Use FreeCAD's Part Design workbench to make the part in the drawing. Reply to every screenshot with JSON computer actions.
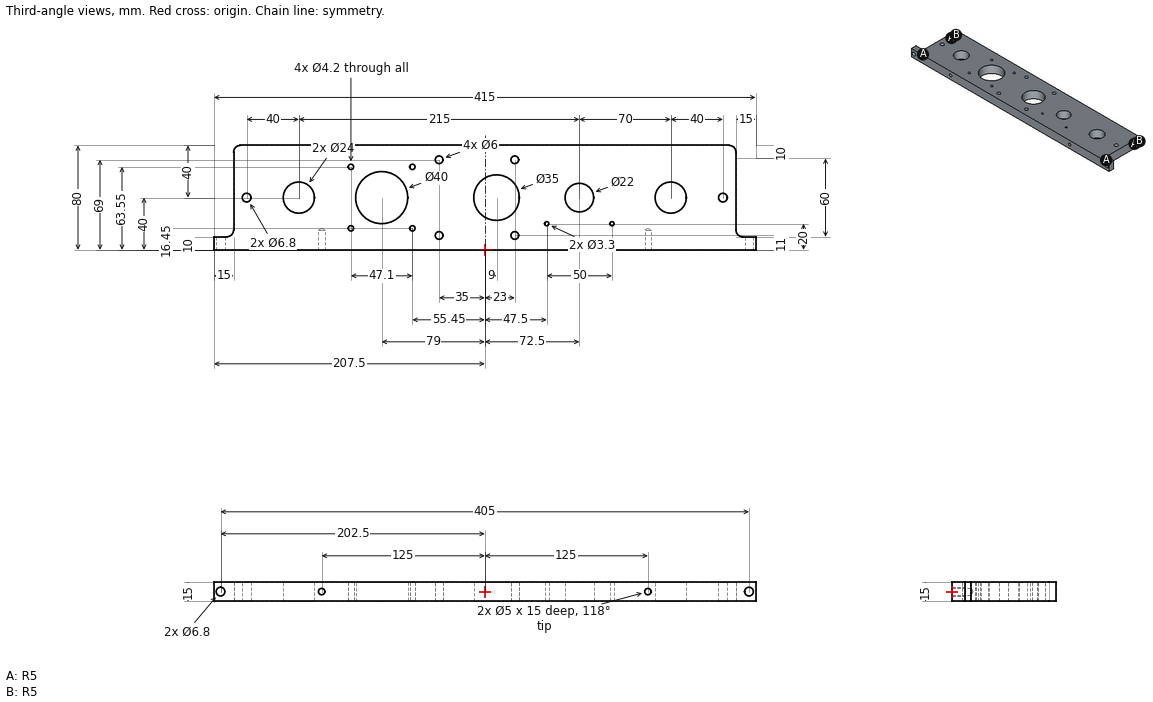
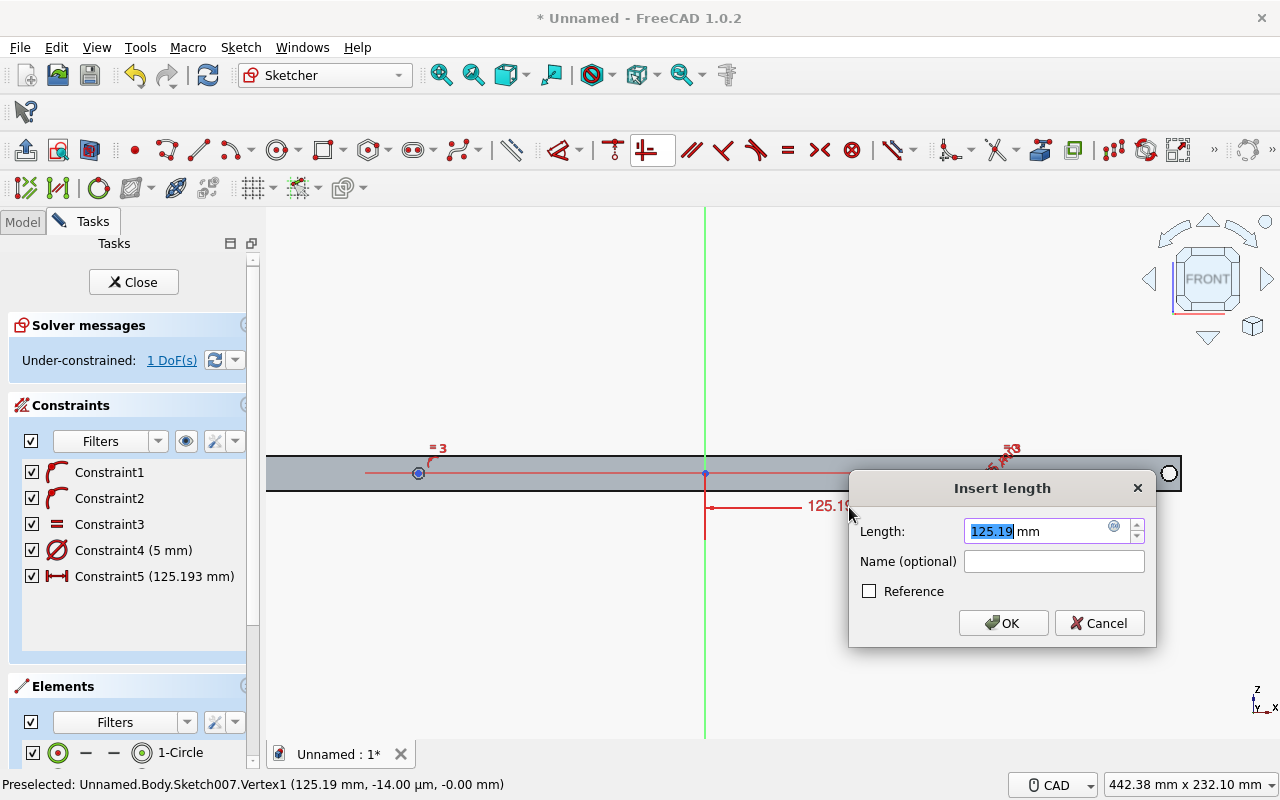
{"action": "type", "text": "125"}
{"action": "key", "text": "Return"}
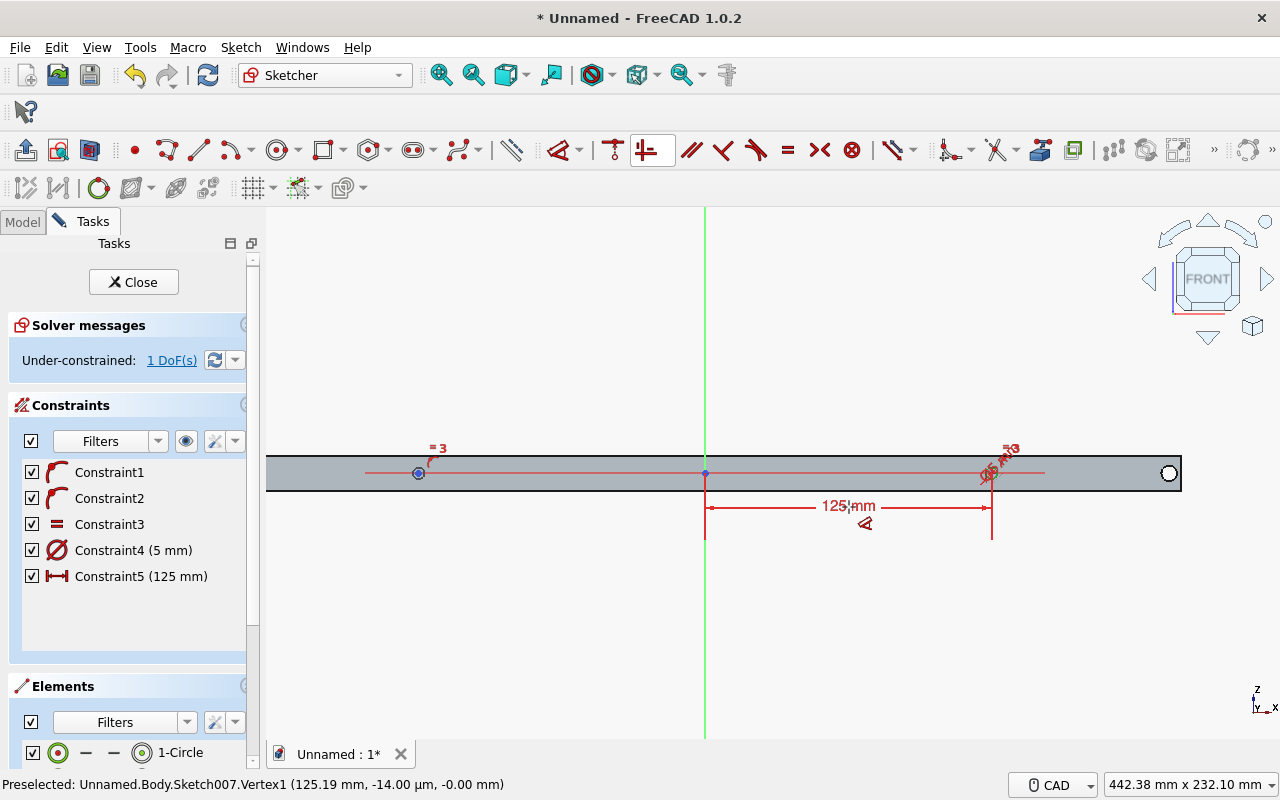
{"action": "left_click", "coordinate": [419, 473]}
{"action": "left_click", "coordinate": [562, 507]}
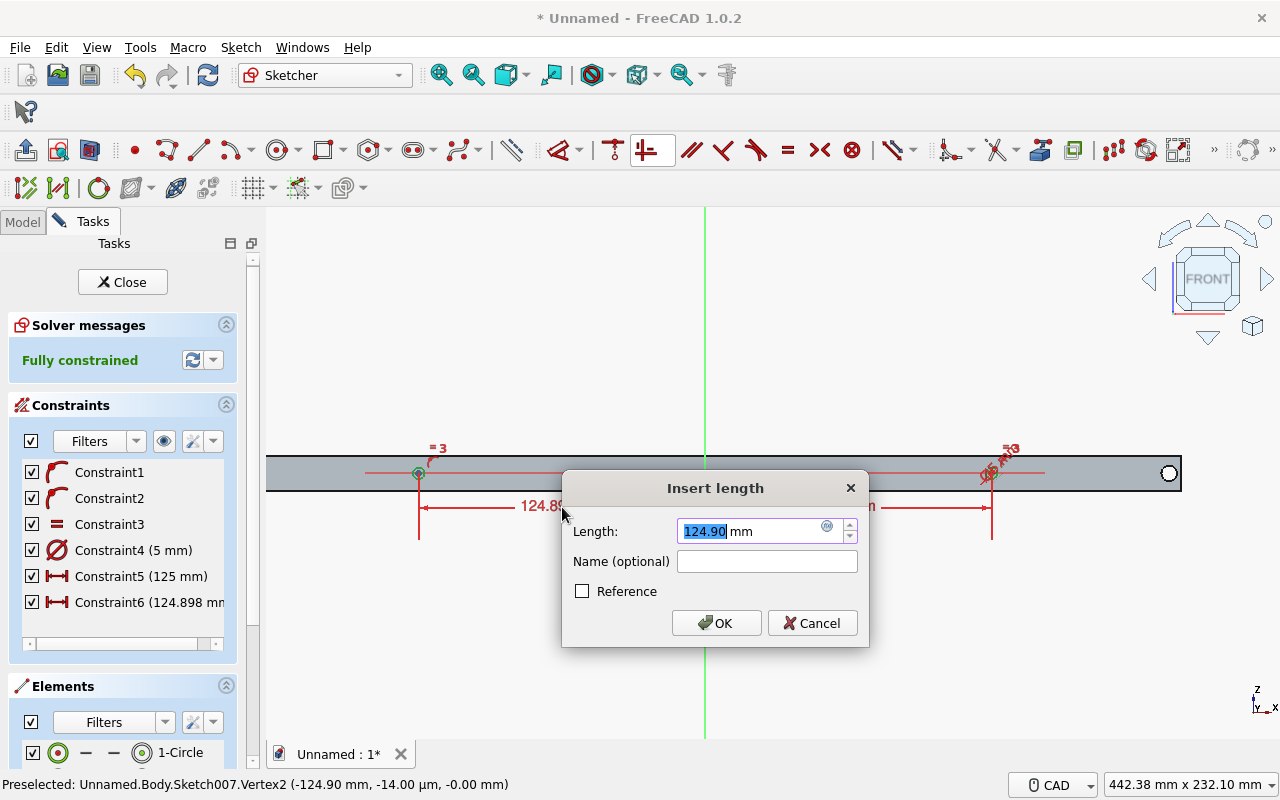
{"action": "type", "text": "125"}
{"action": "key", "text": "Return"}
{"action": "key", "text": "Escape"}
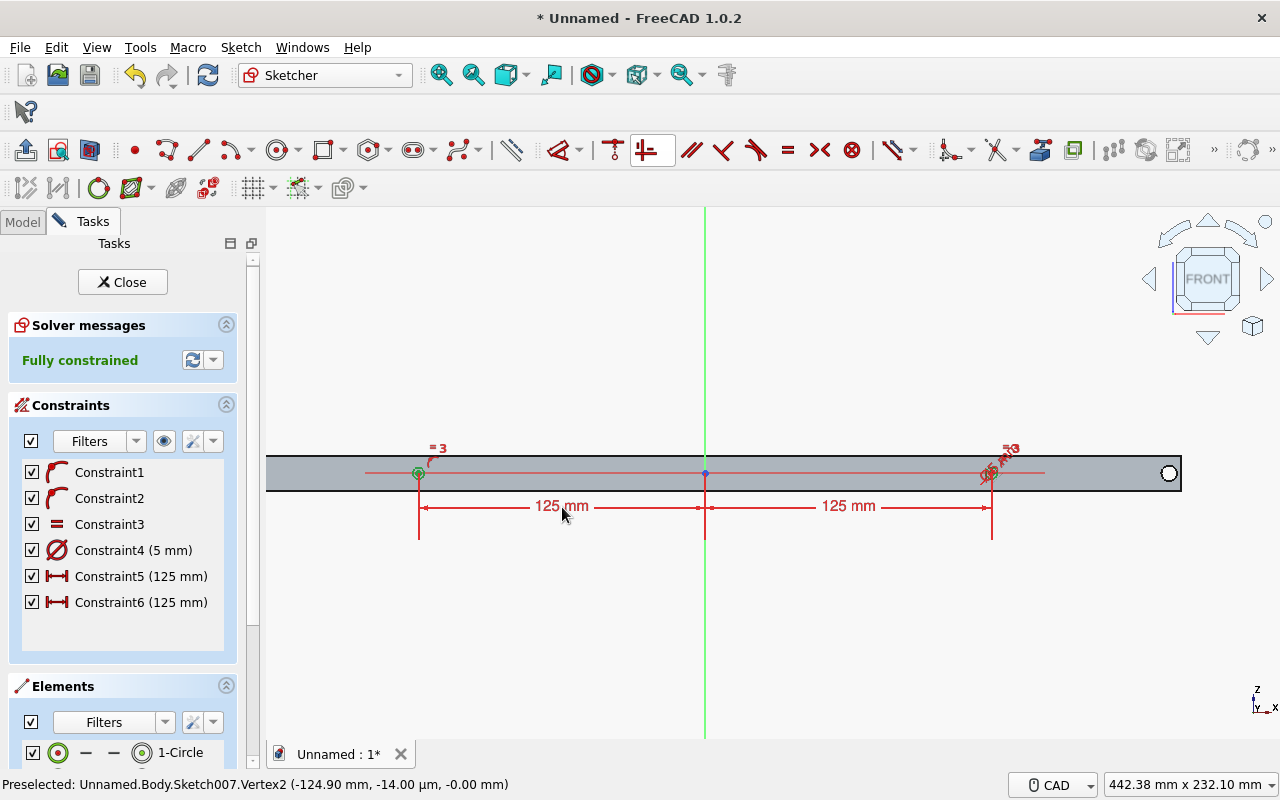
{"action": "left_click", "coordinate": [123, 282]}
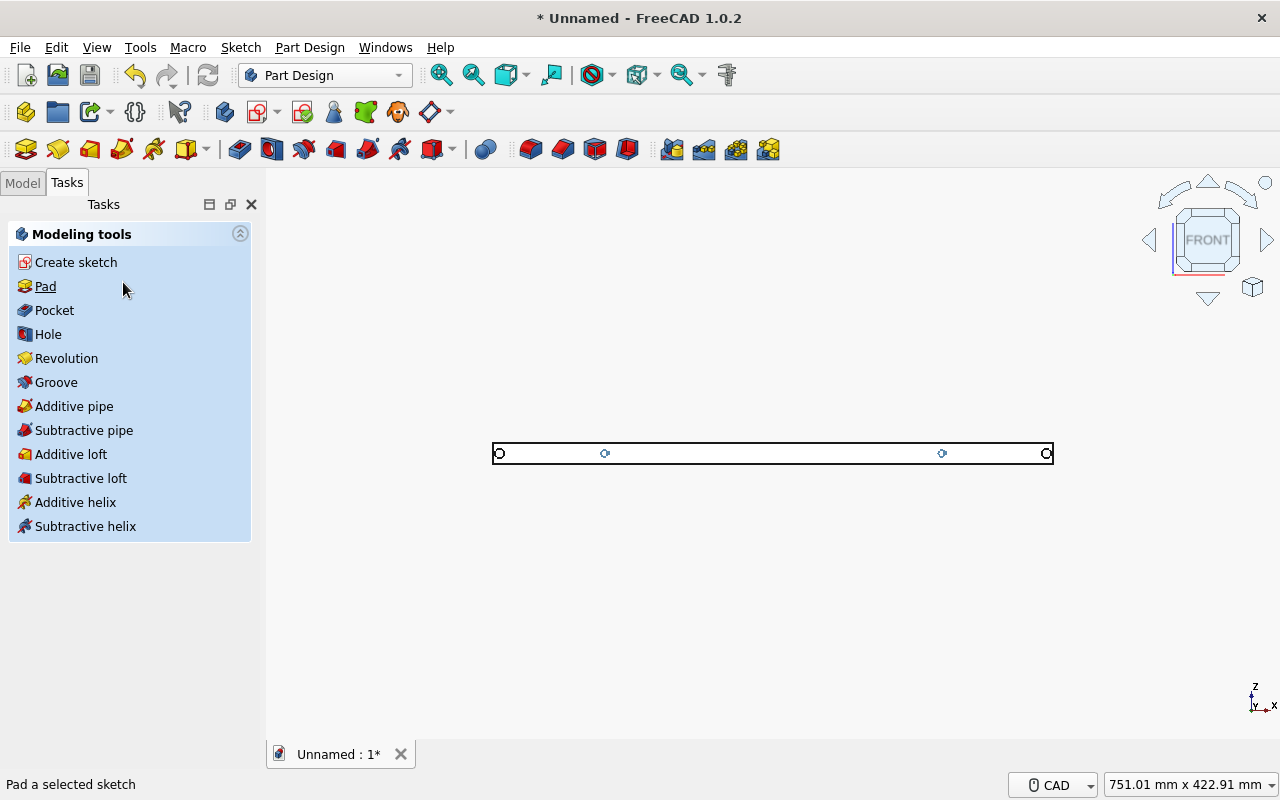
{"action": "left_click", "coordinate": [272, 150]}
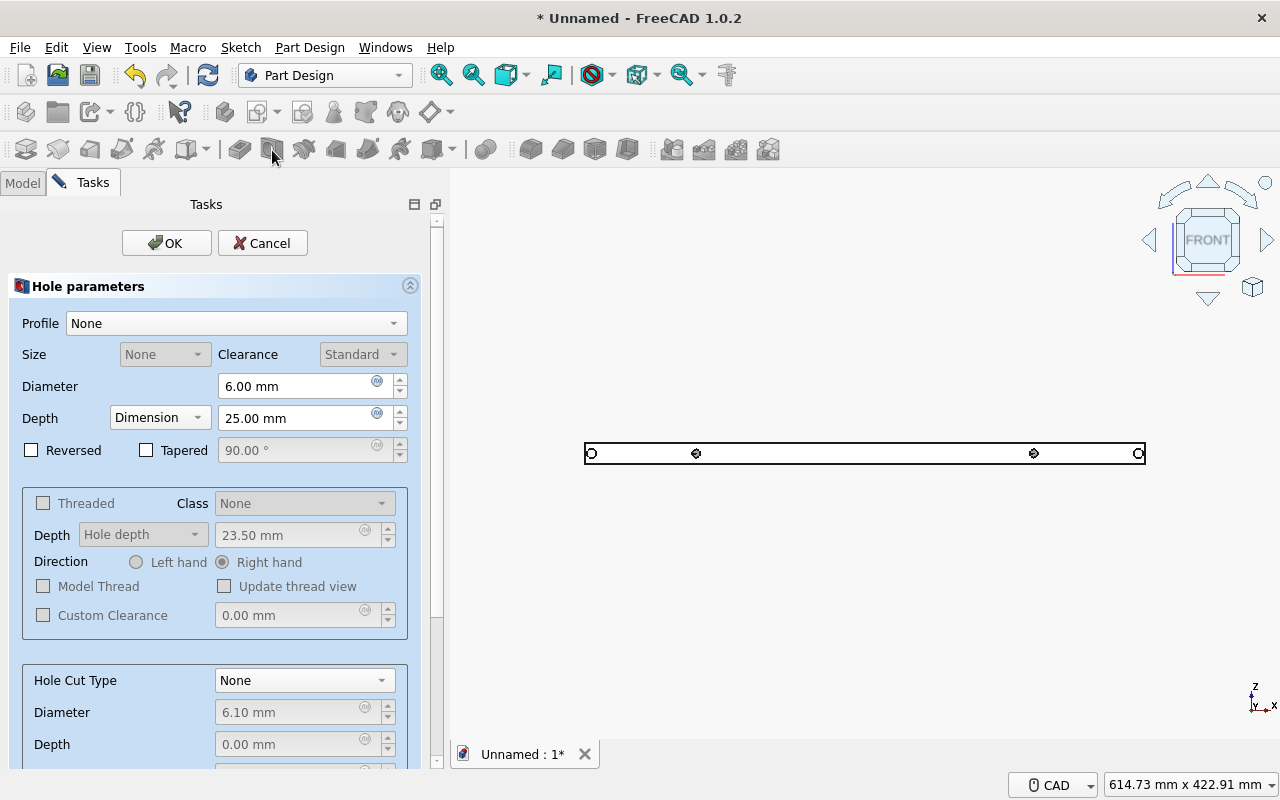
{"action": "triple_click", "coordinate": [305, 386]}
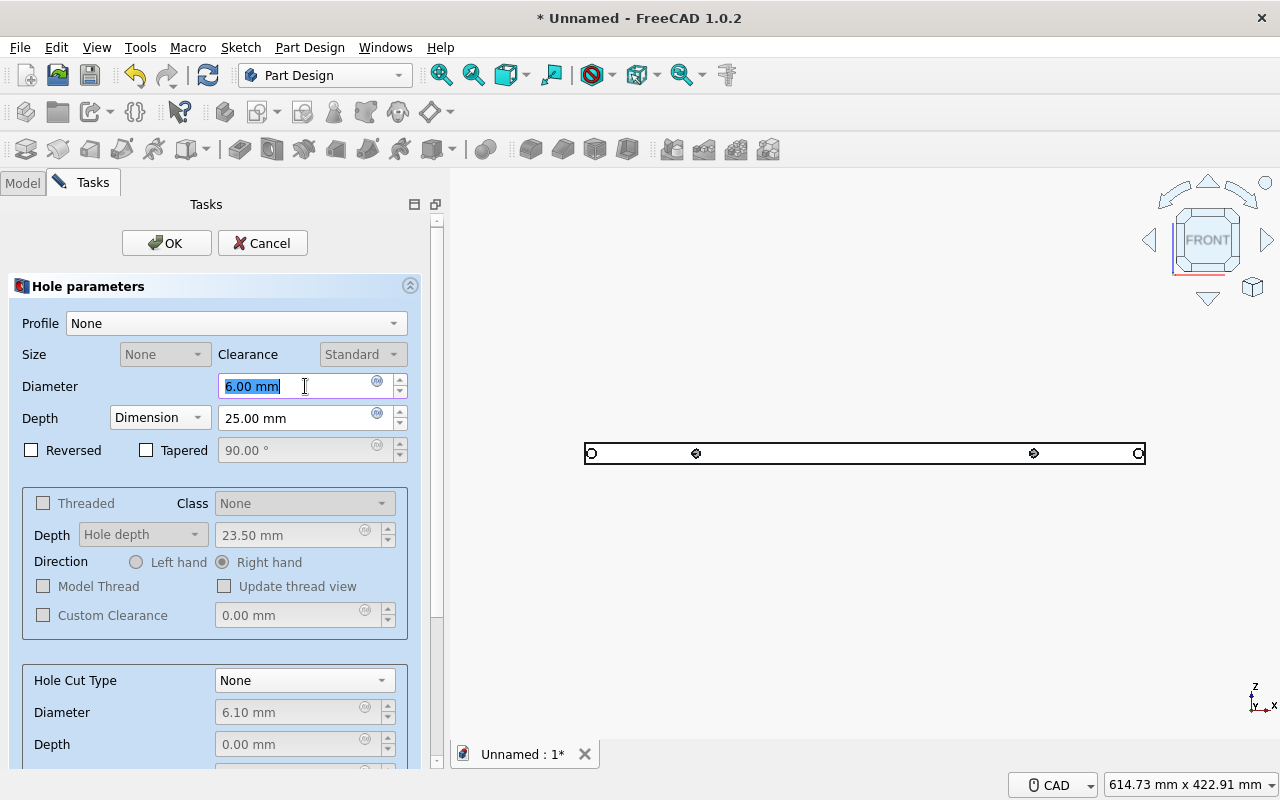
{"action": "type", "text": "5"}
{"action": "key", "text": "Tab"}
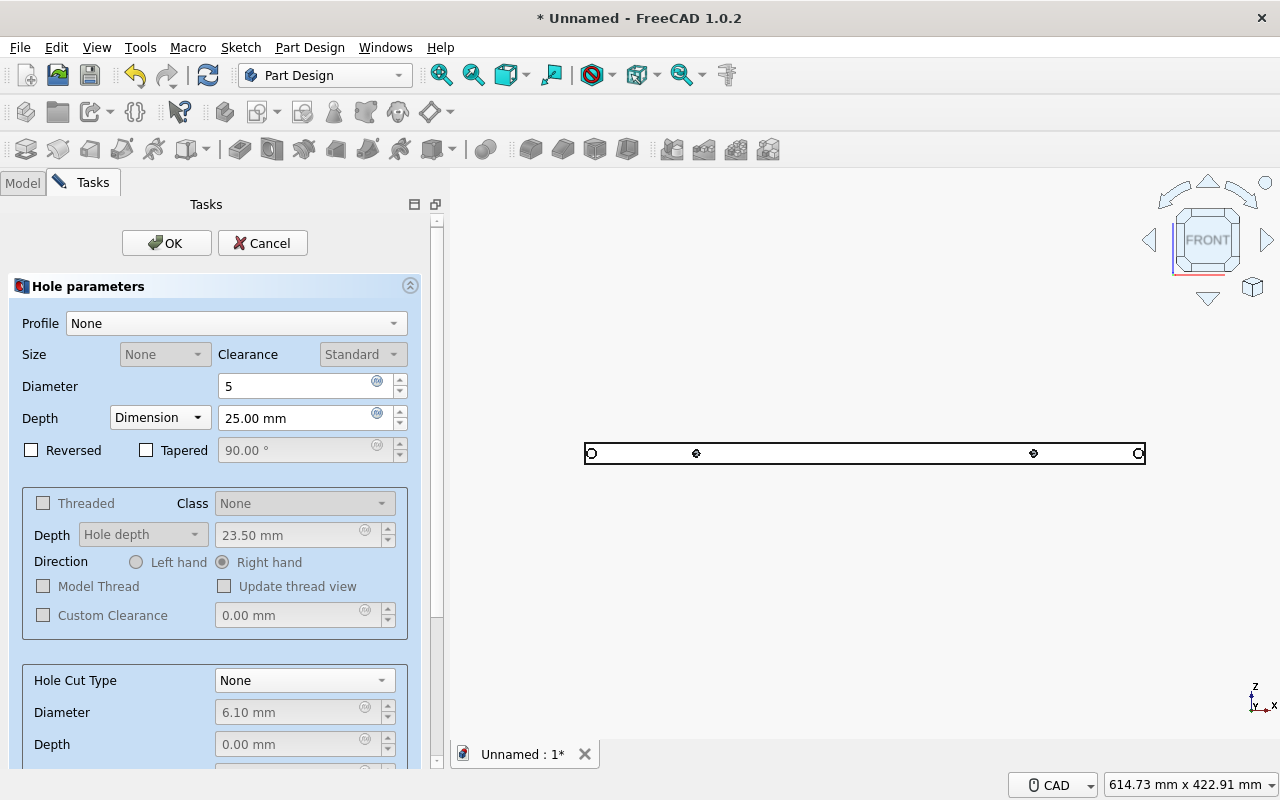
{"action": "triple_click", "coordinate": [305, 418]}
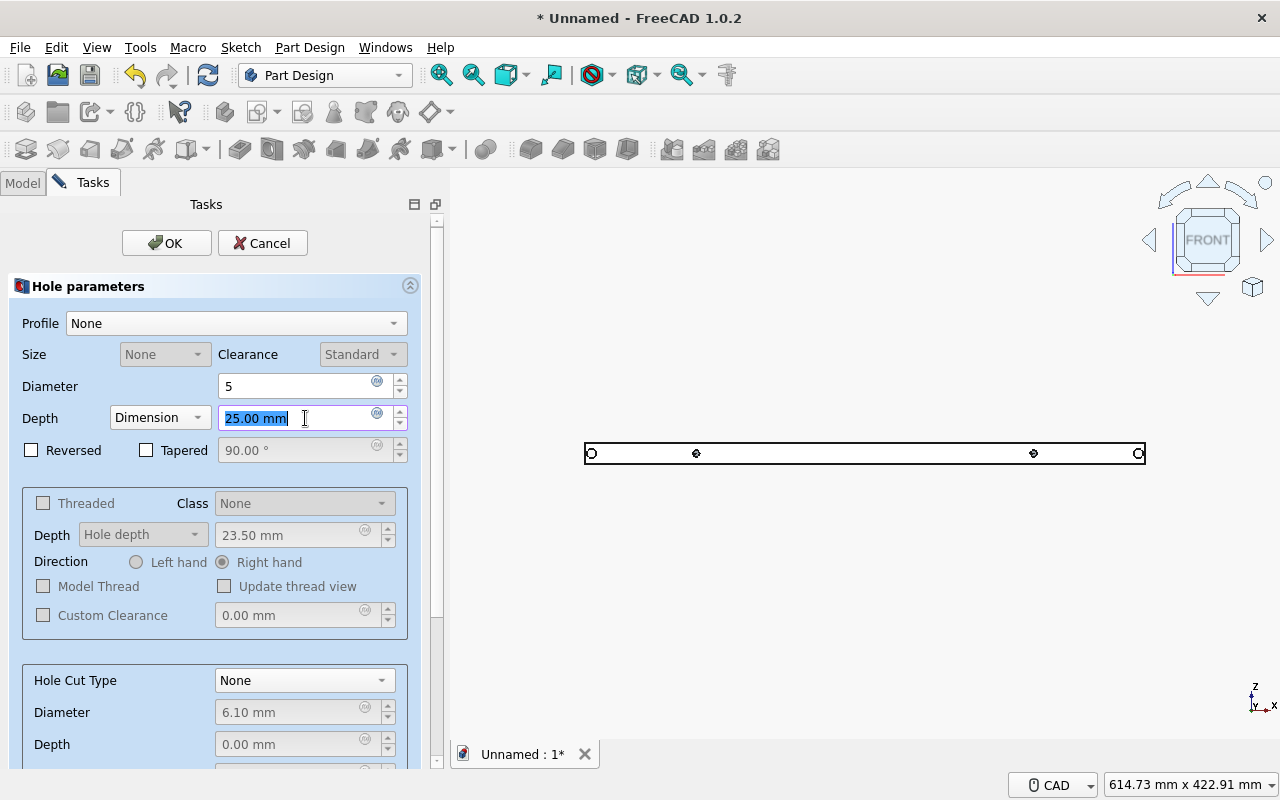
{"action": "type", "text": "15"}
{"action": "key", "text": "Tab"}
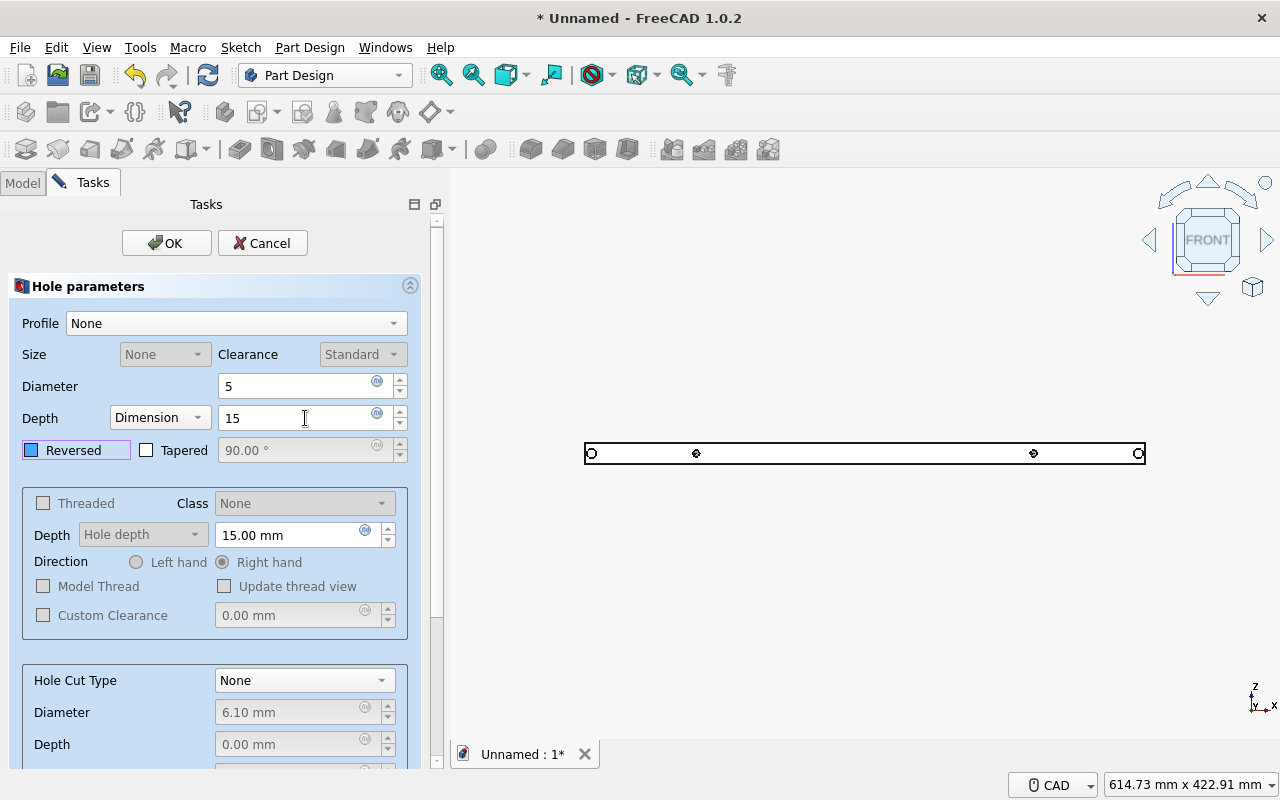
{"action": "left_click", "coordinate": [167, 243]}